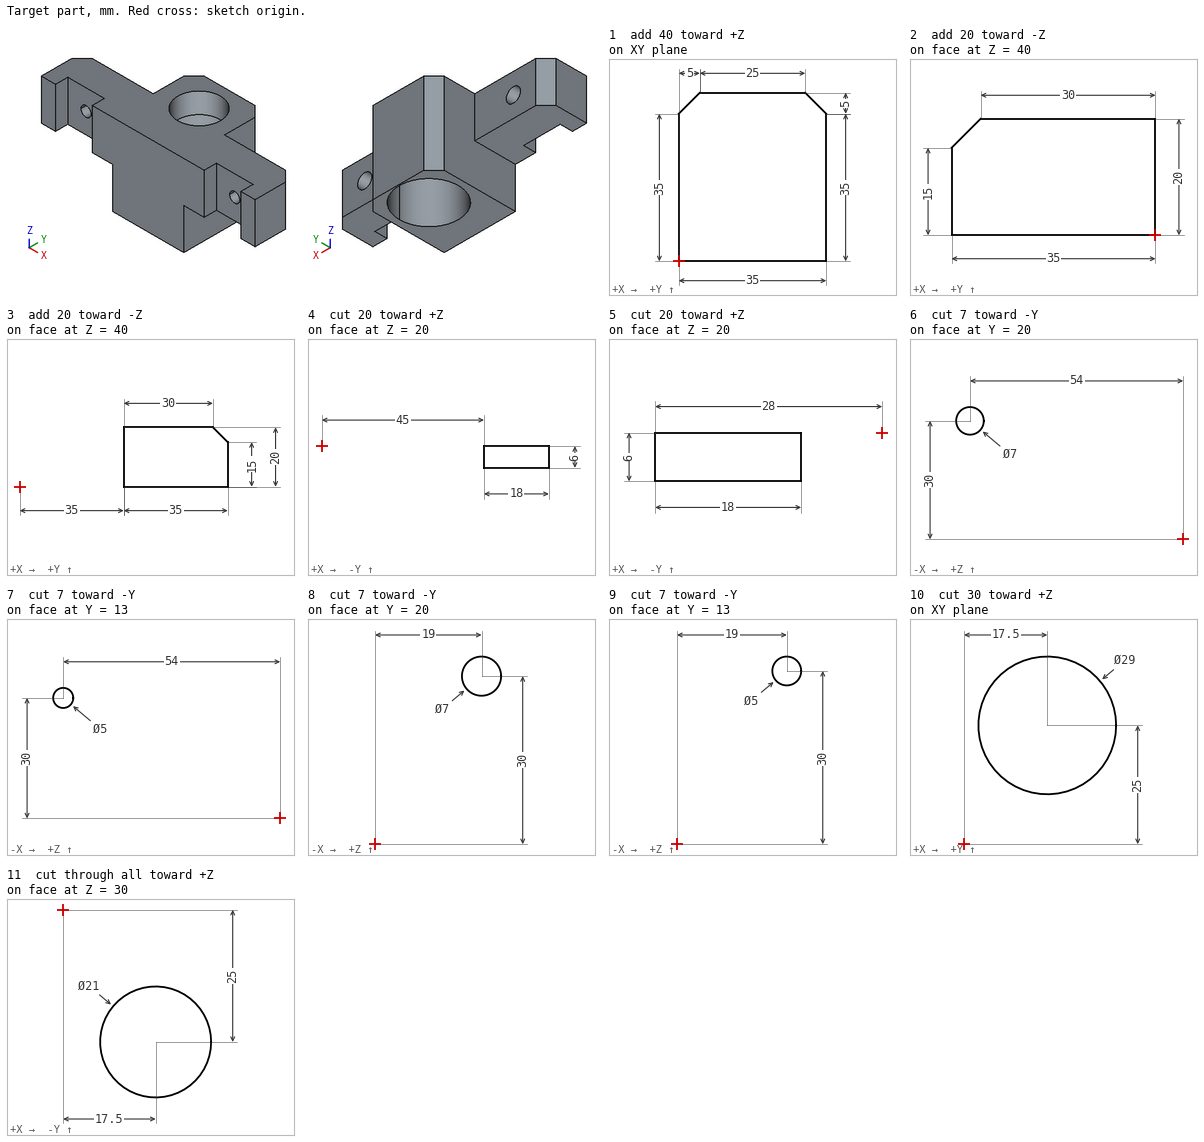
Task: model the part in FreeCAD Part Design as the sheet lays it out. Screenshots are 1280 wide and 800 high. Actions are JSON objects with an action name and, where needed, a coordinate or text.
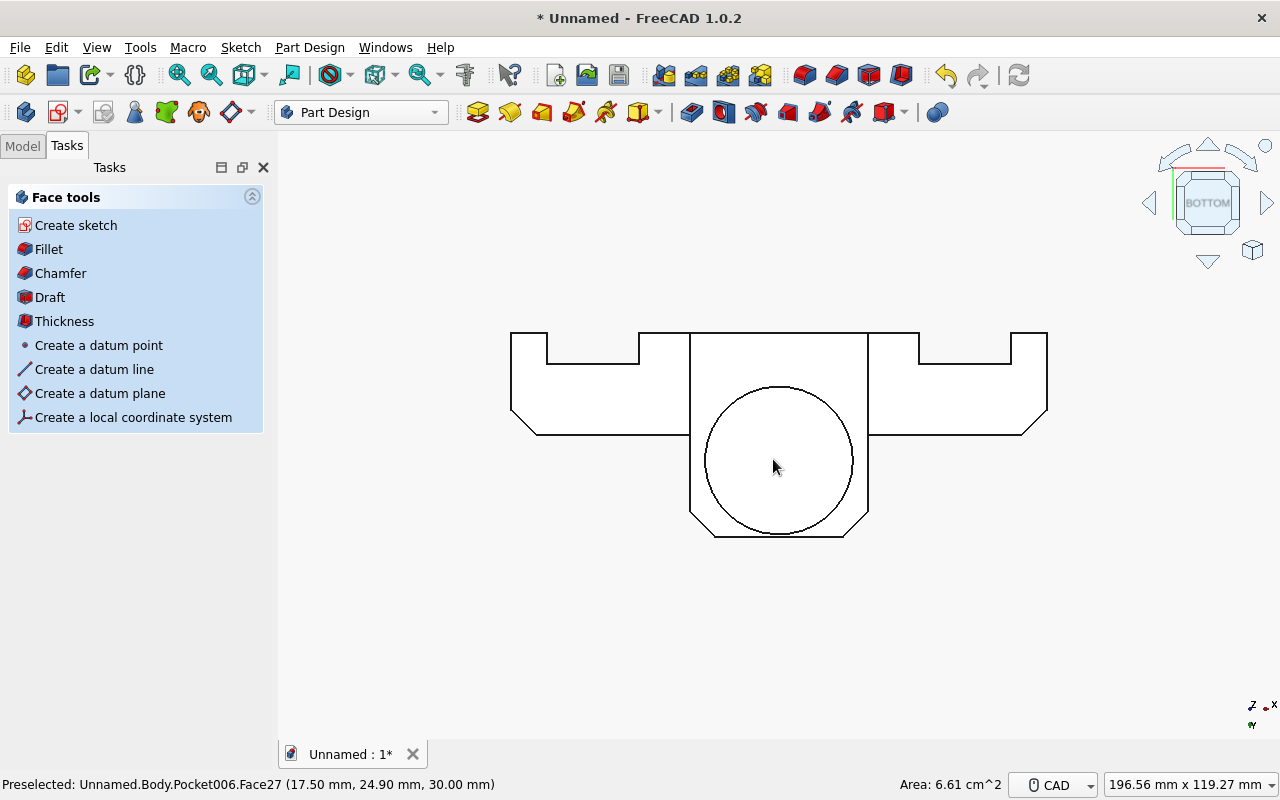
{"action": "left_click", "coordinate": [58, 112]}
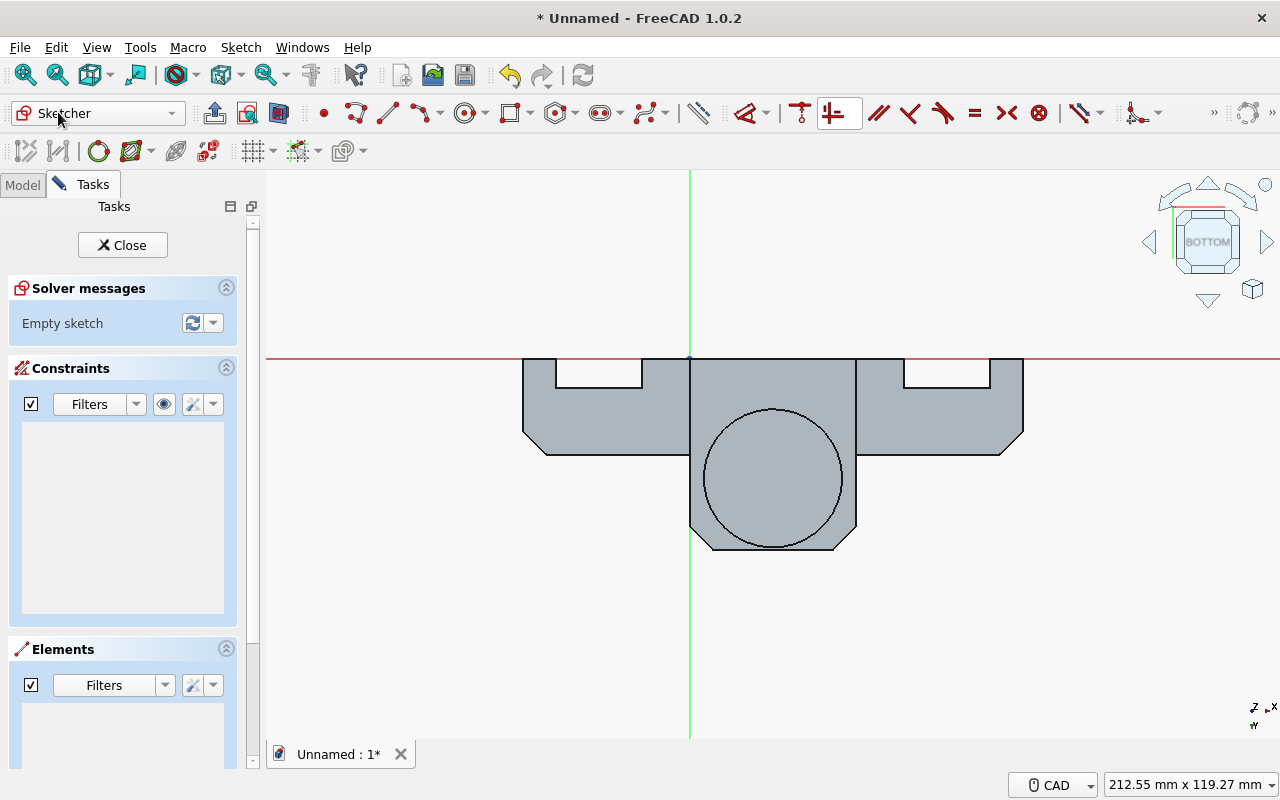
{"action": "scroll", "coordinate": [799, 435], "scroll_direction": "up", "scroll_amount": 4}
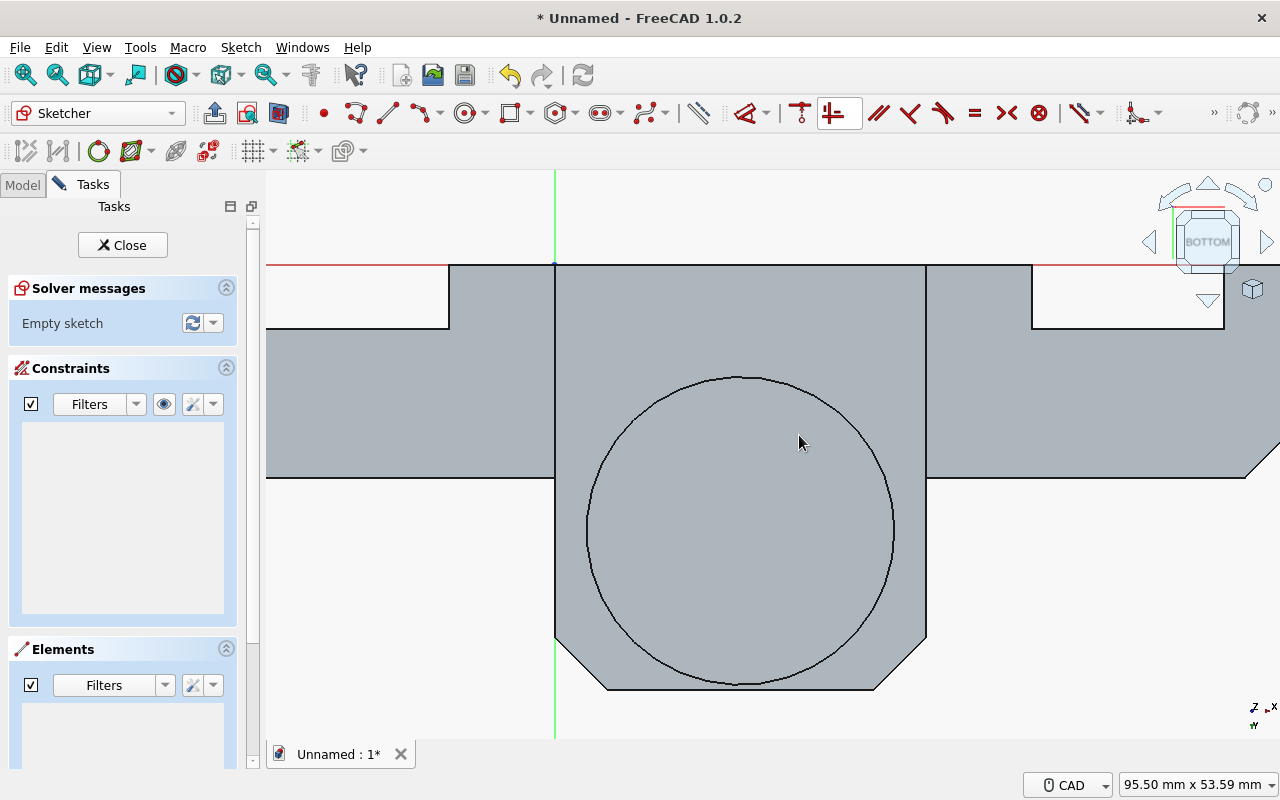
{"action": "left_click", "coordinate": [466, 114]}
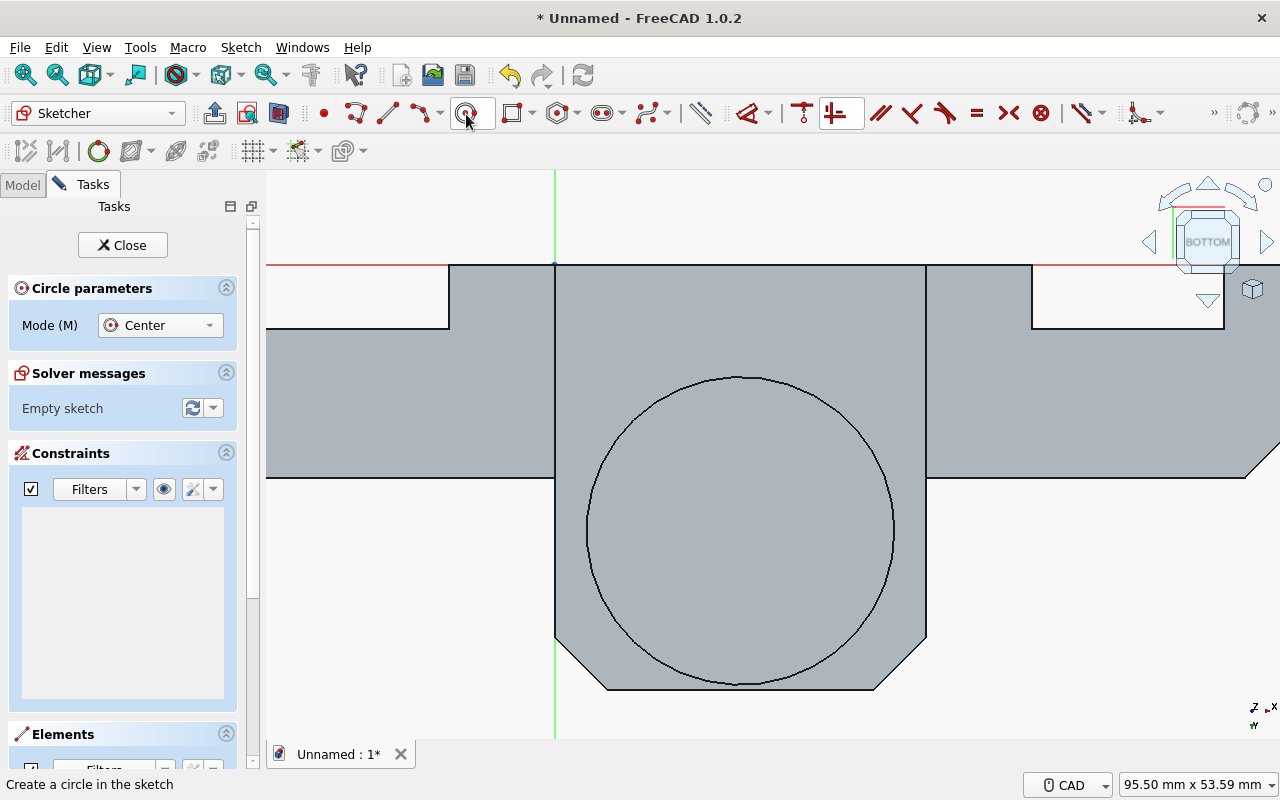
{"action": "left_click", "coordinate": [740, 531]}
{"action": "left_click", "coordinate": [819, 452]}
{"action": "key", "text": "Escape"}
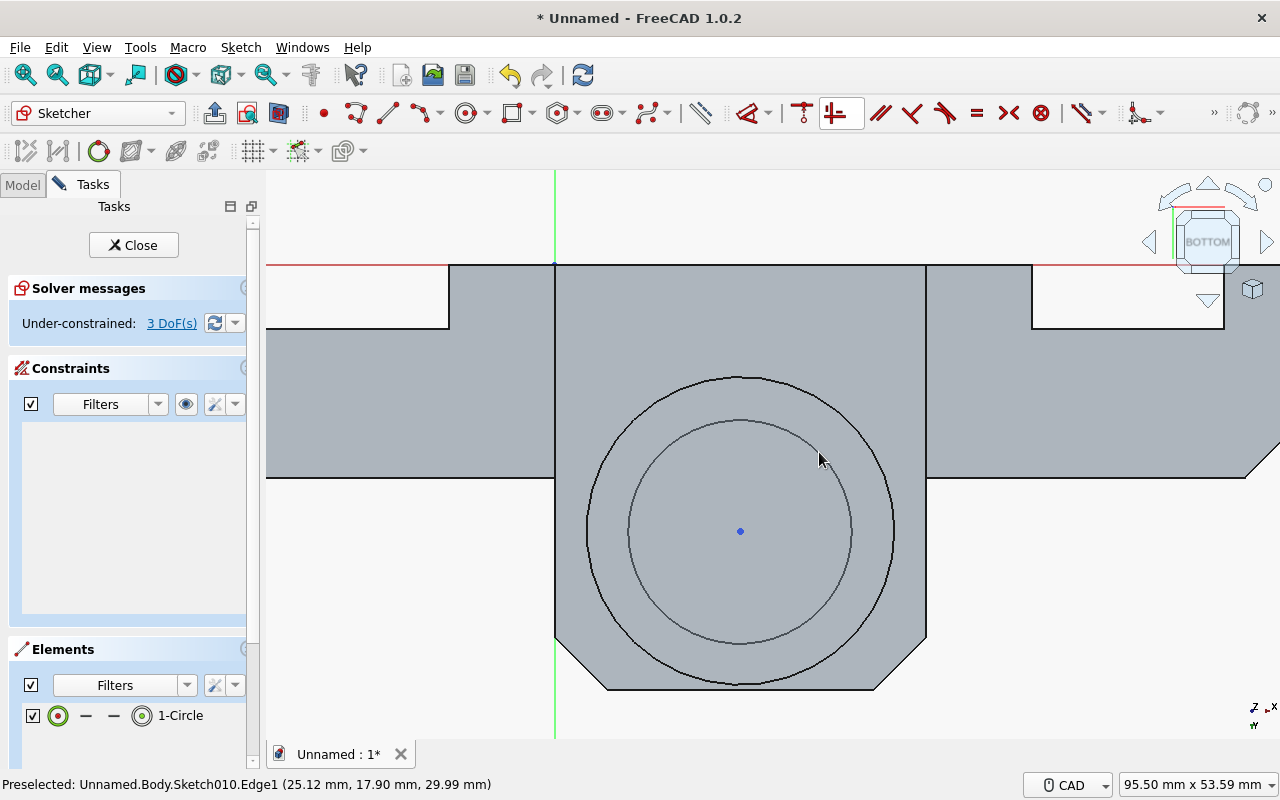
{"action": "left_click", "coordinate": [748, 114]}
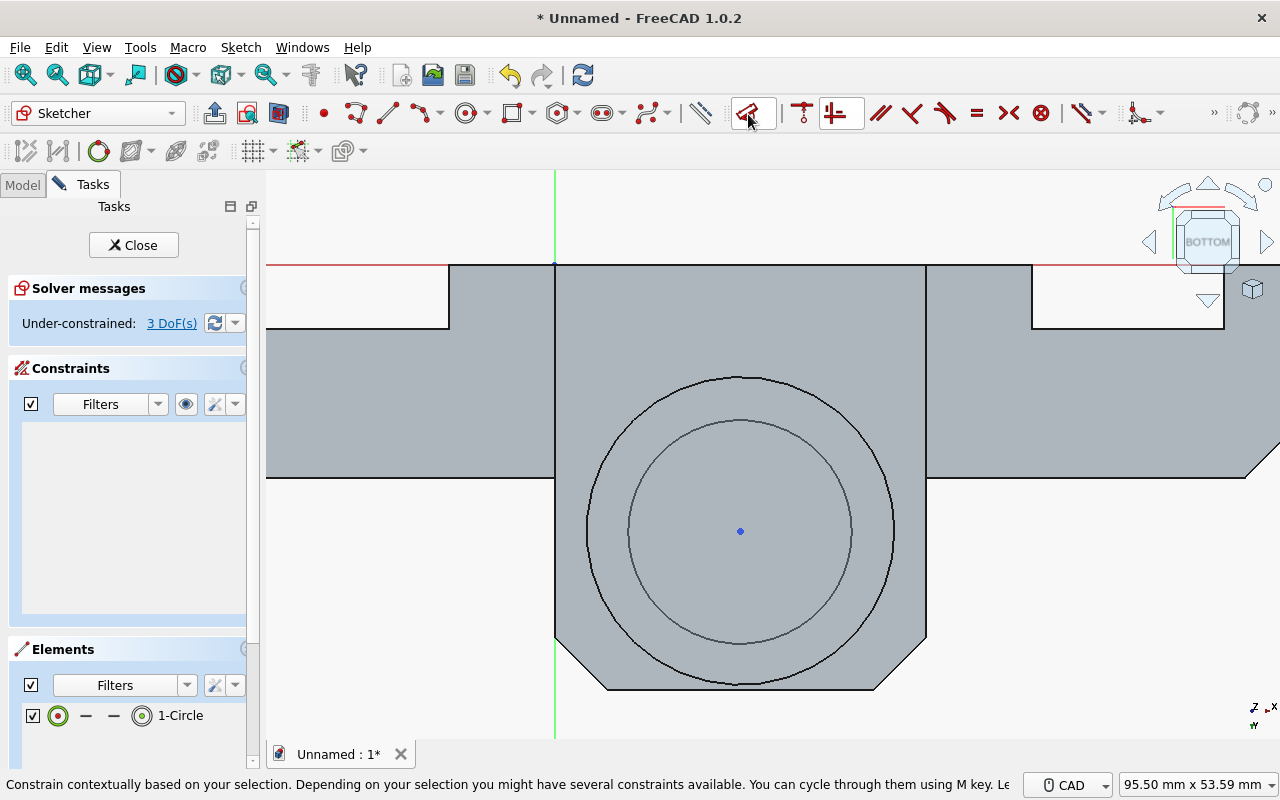
{"action": "left_click", "coordinate": [819, 453]}
{"action": "left_click", "coordinate": [842, 430]}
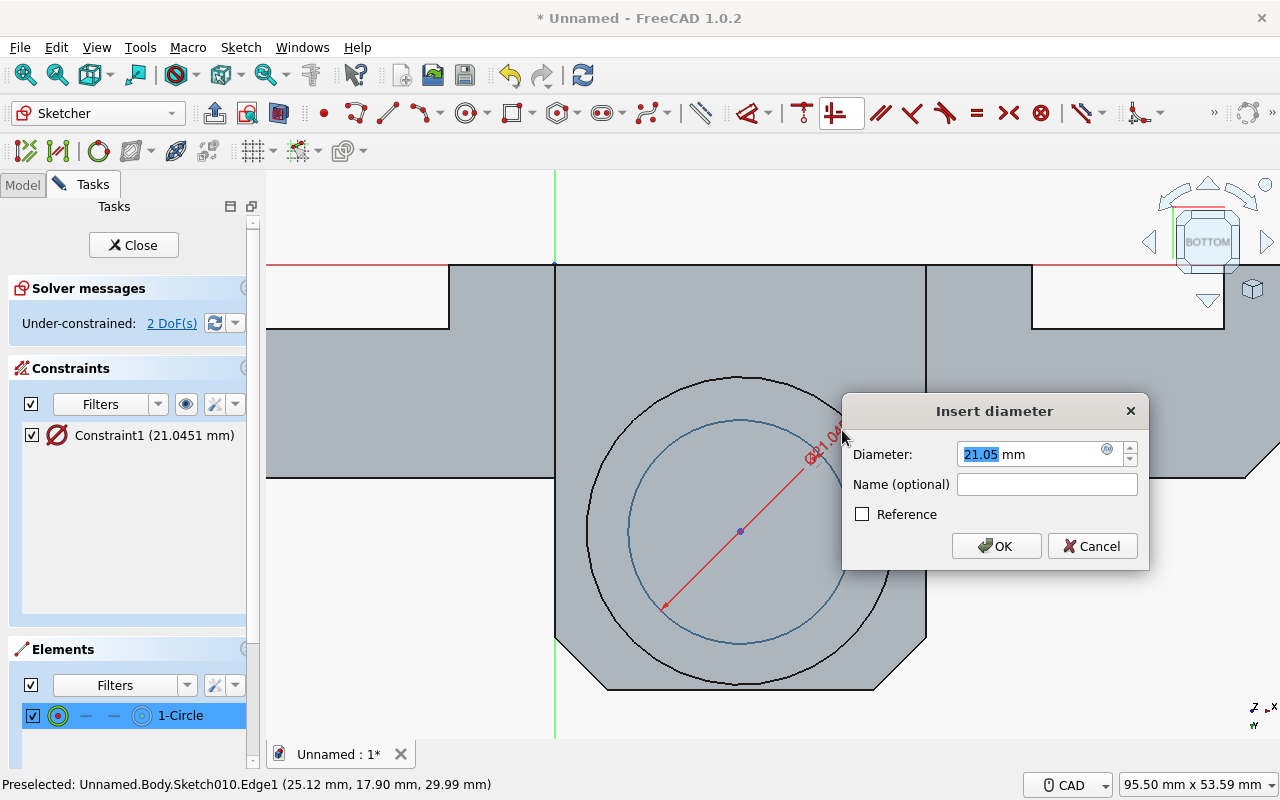
{"action": "type", "text": "21"}
{"action": "key", "text": "Return"}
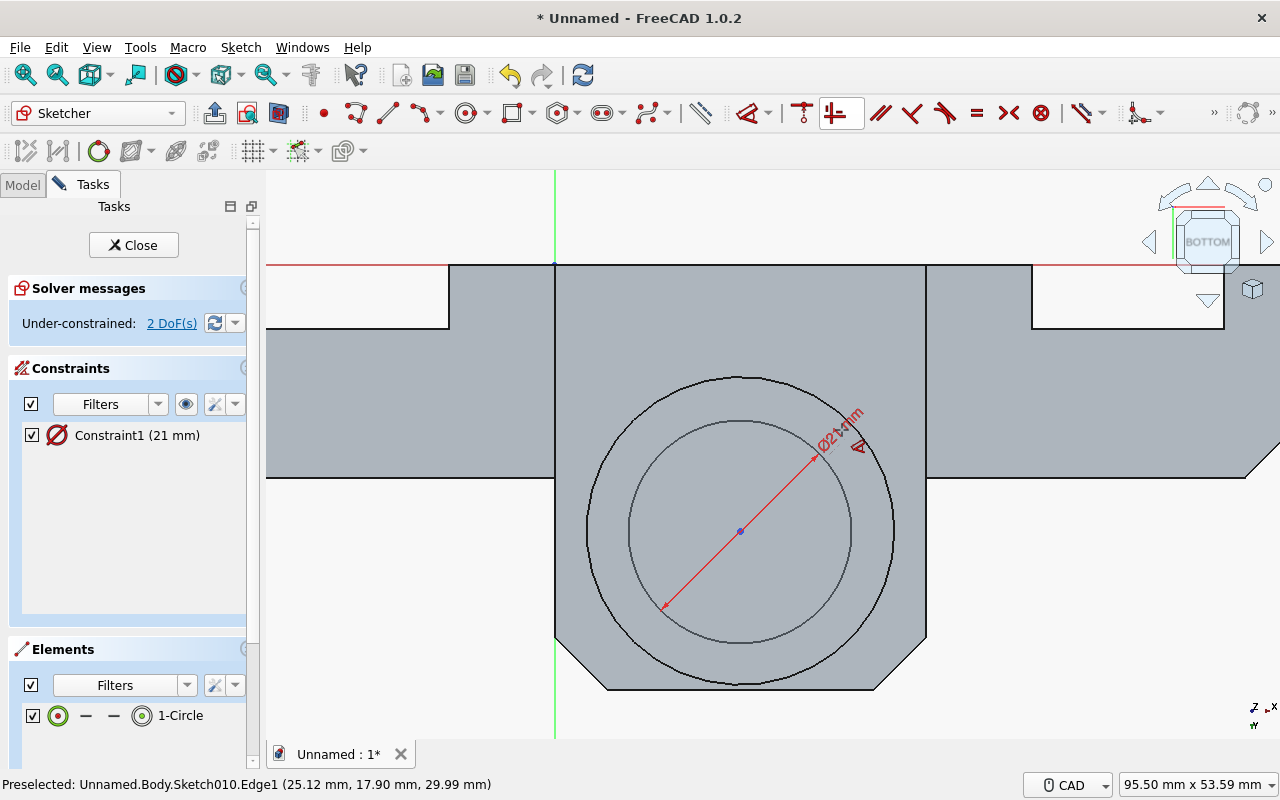
{"action": "left_click", "coordinate": [740, 532]}
{"action": "left_click", "coordinate": [521, 399]}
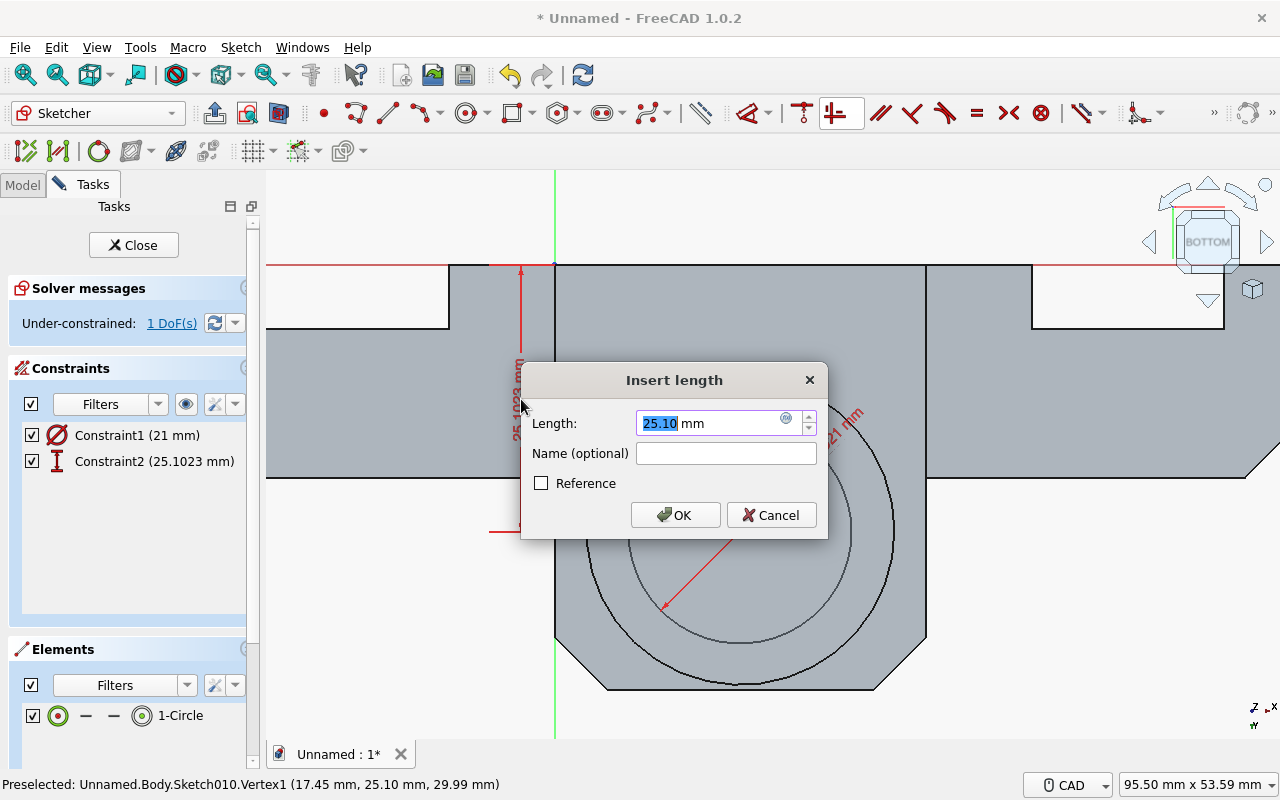
{"action": "type", "text": "25"}
{"action": "key", "text": "Return"}